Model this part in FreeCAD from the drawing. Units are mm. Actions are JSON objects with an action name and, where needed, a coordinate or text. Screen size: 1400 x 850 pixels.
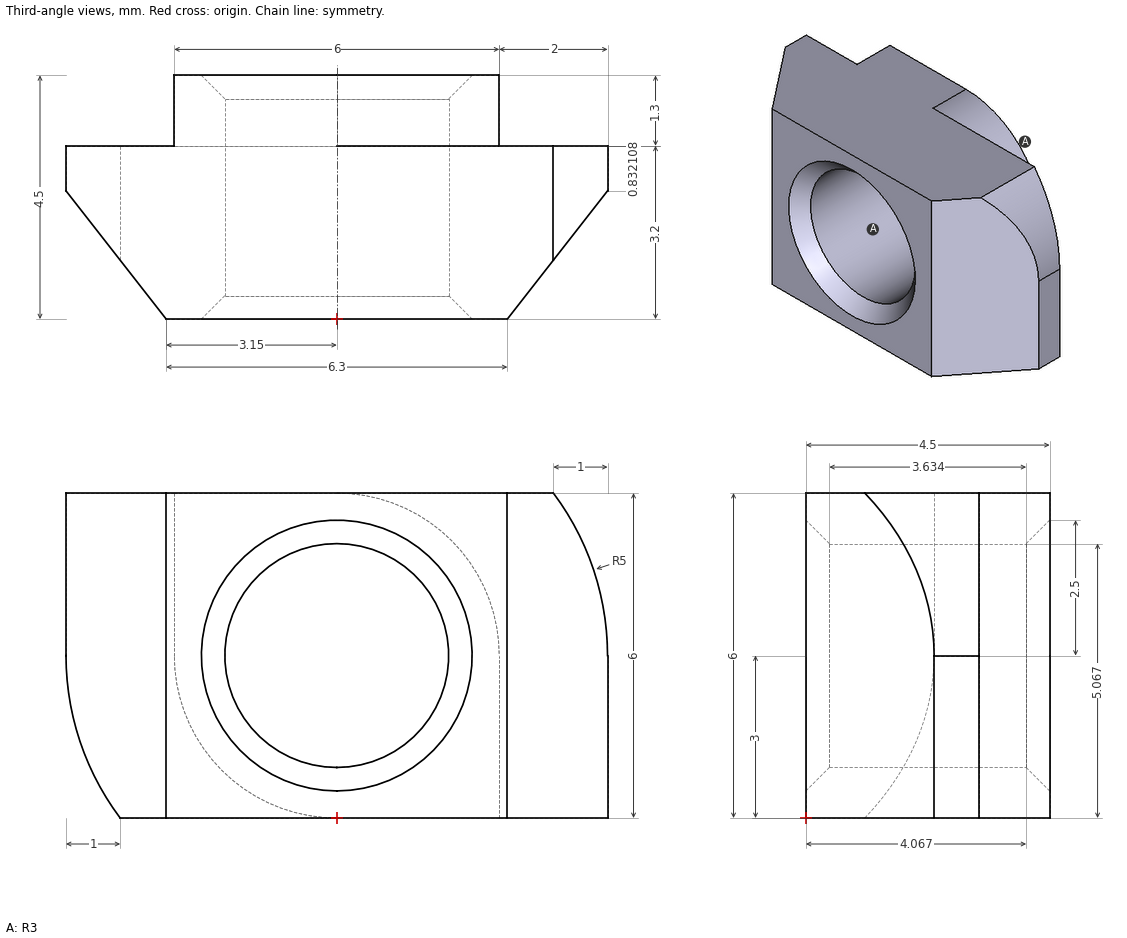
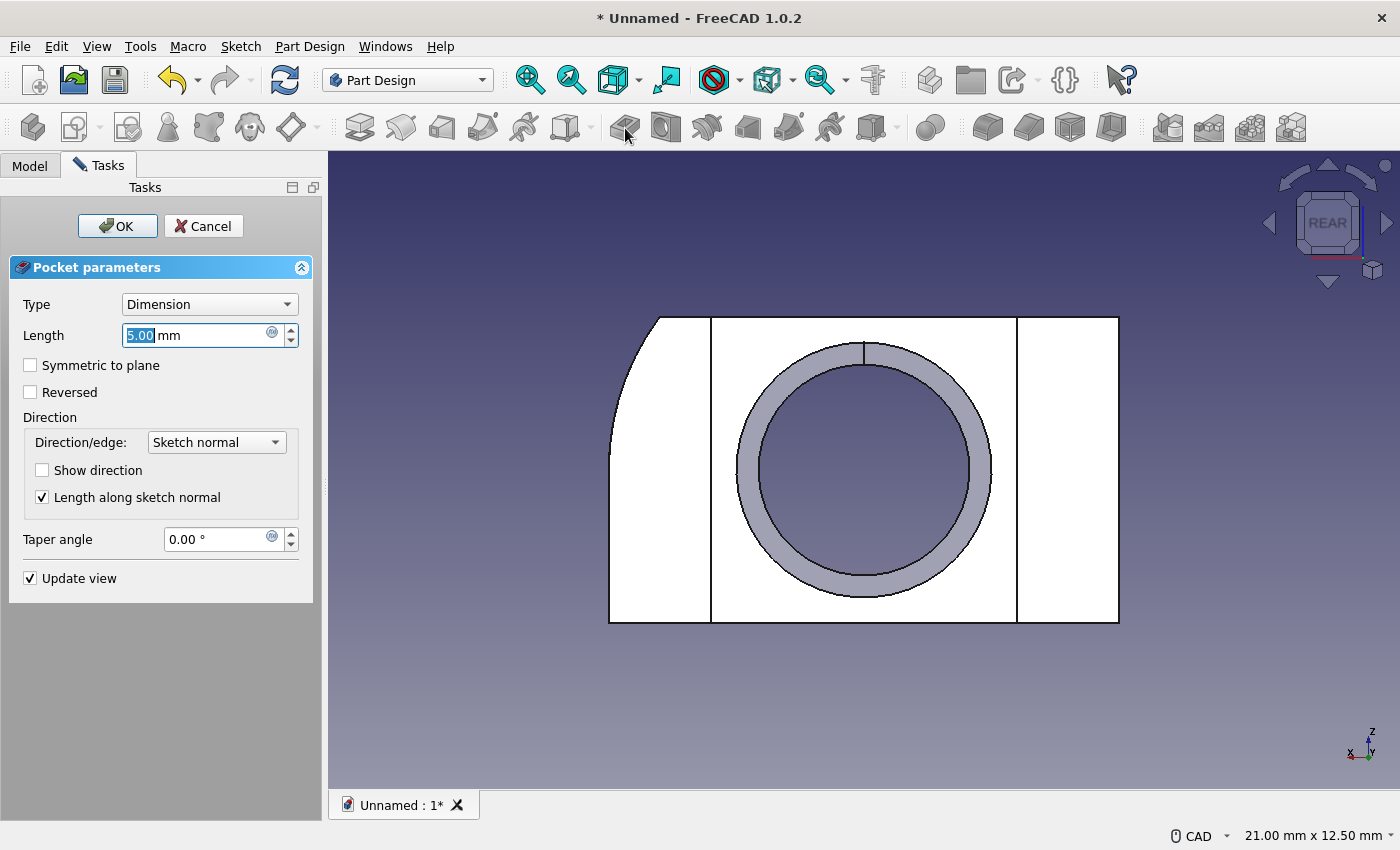
{"action": "type", "text": "4.5"}
{"action": "key", "text": "Tab"}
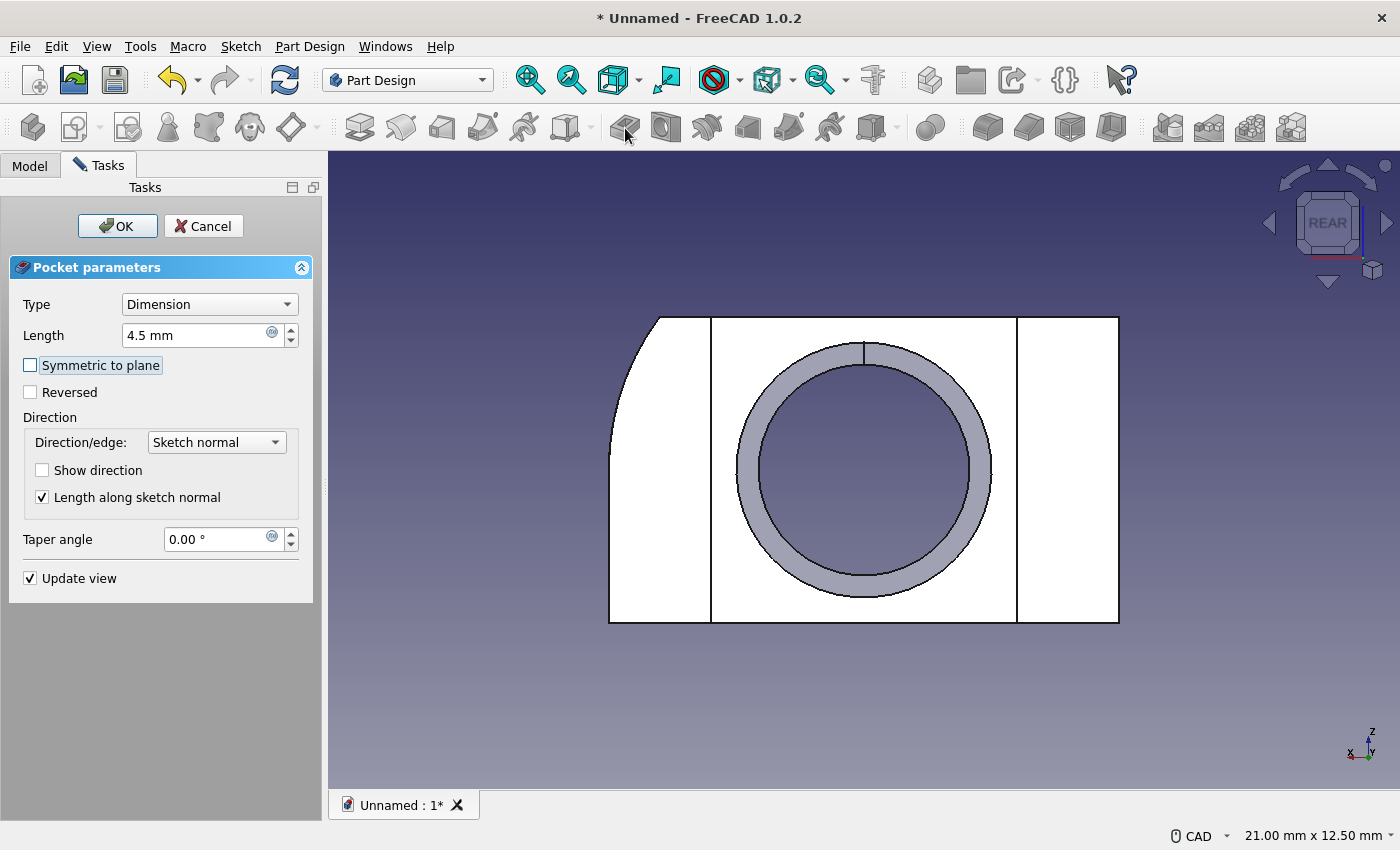
{"action": "left_click", "coordinate": [118, 226]}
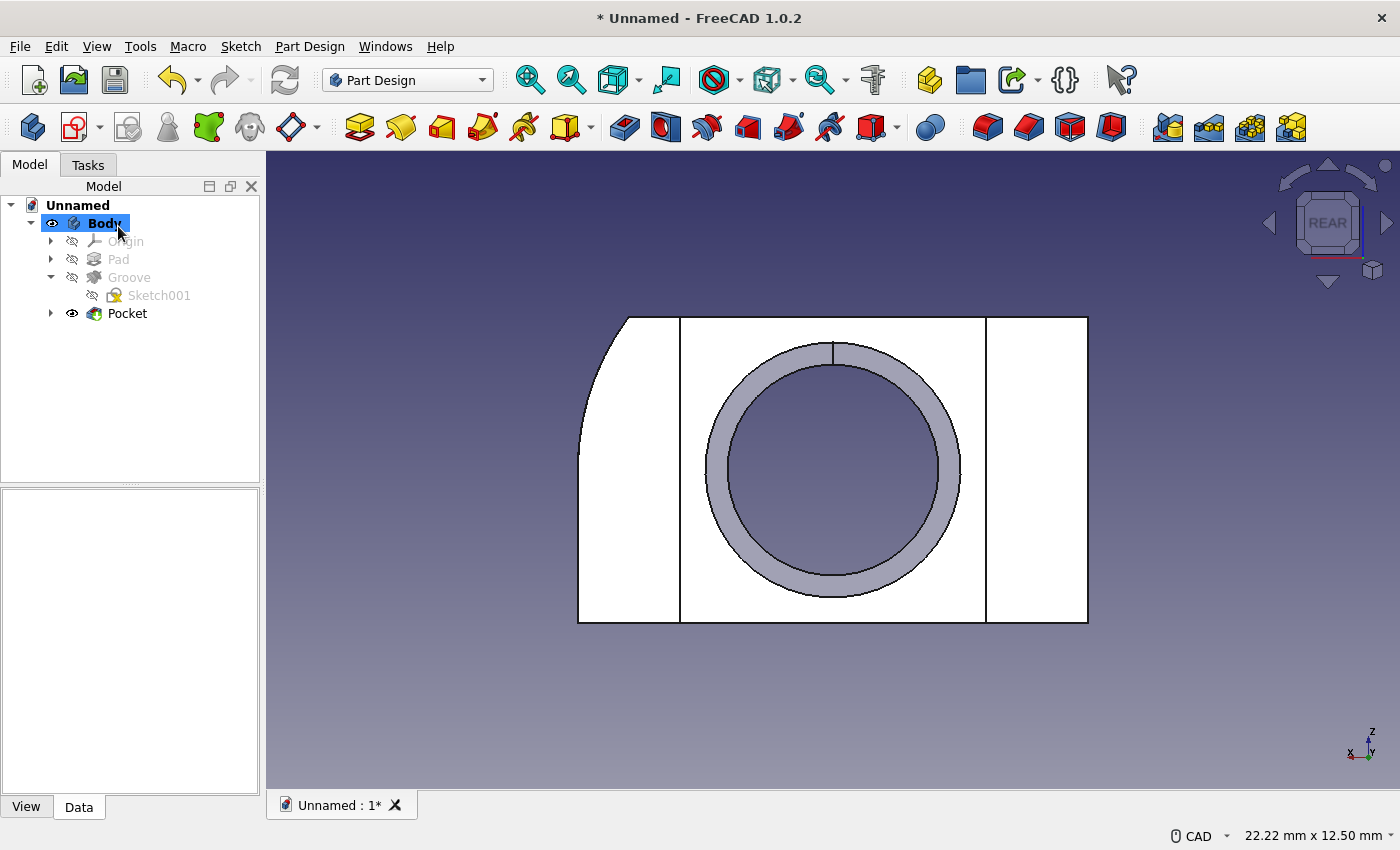
{"action": "left_click", "coordinate": [746, 338]}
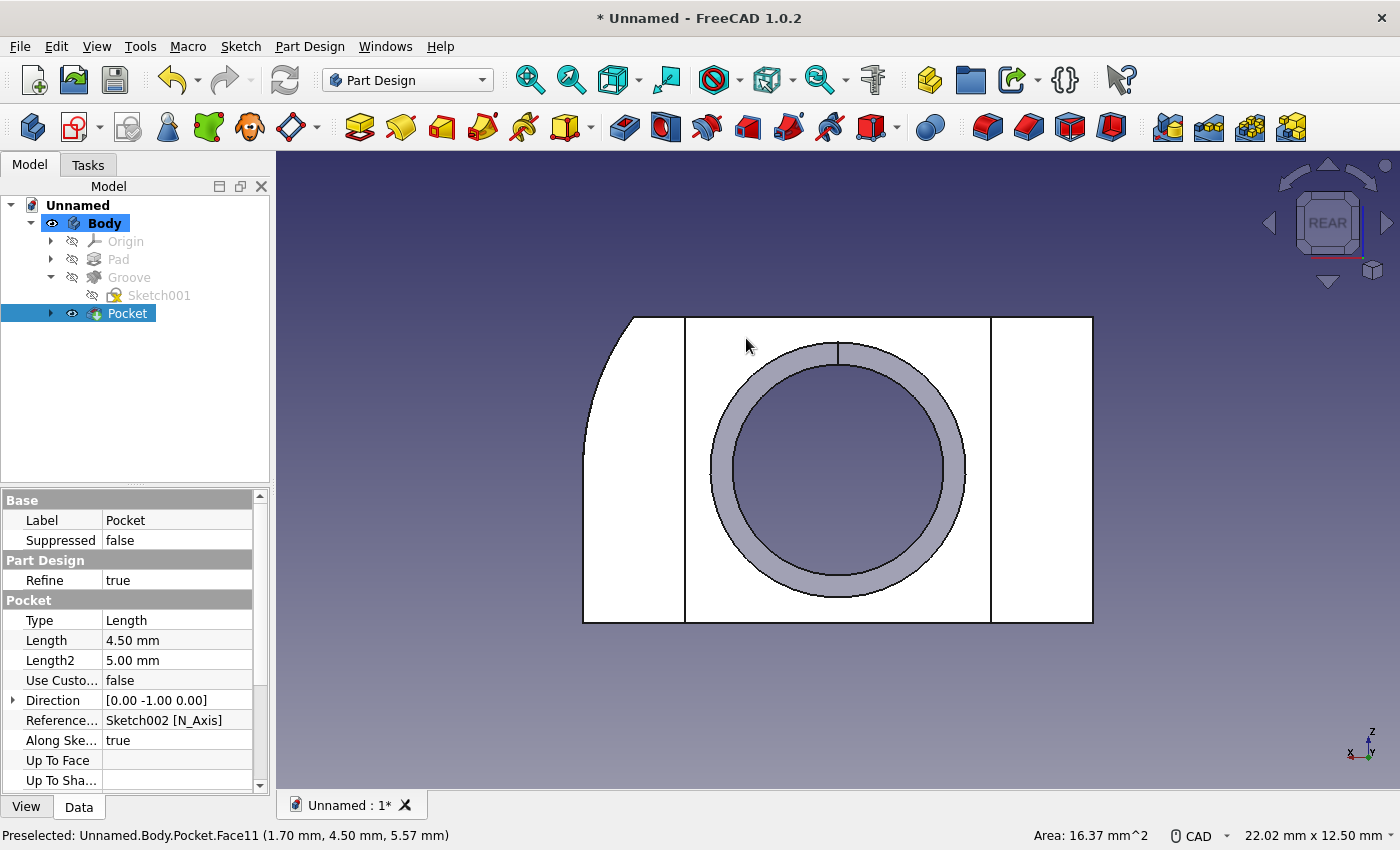
{"action": "left_click", "coordinate": [74, 128]}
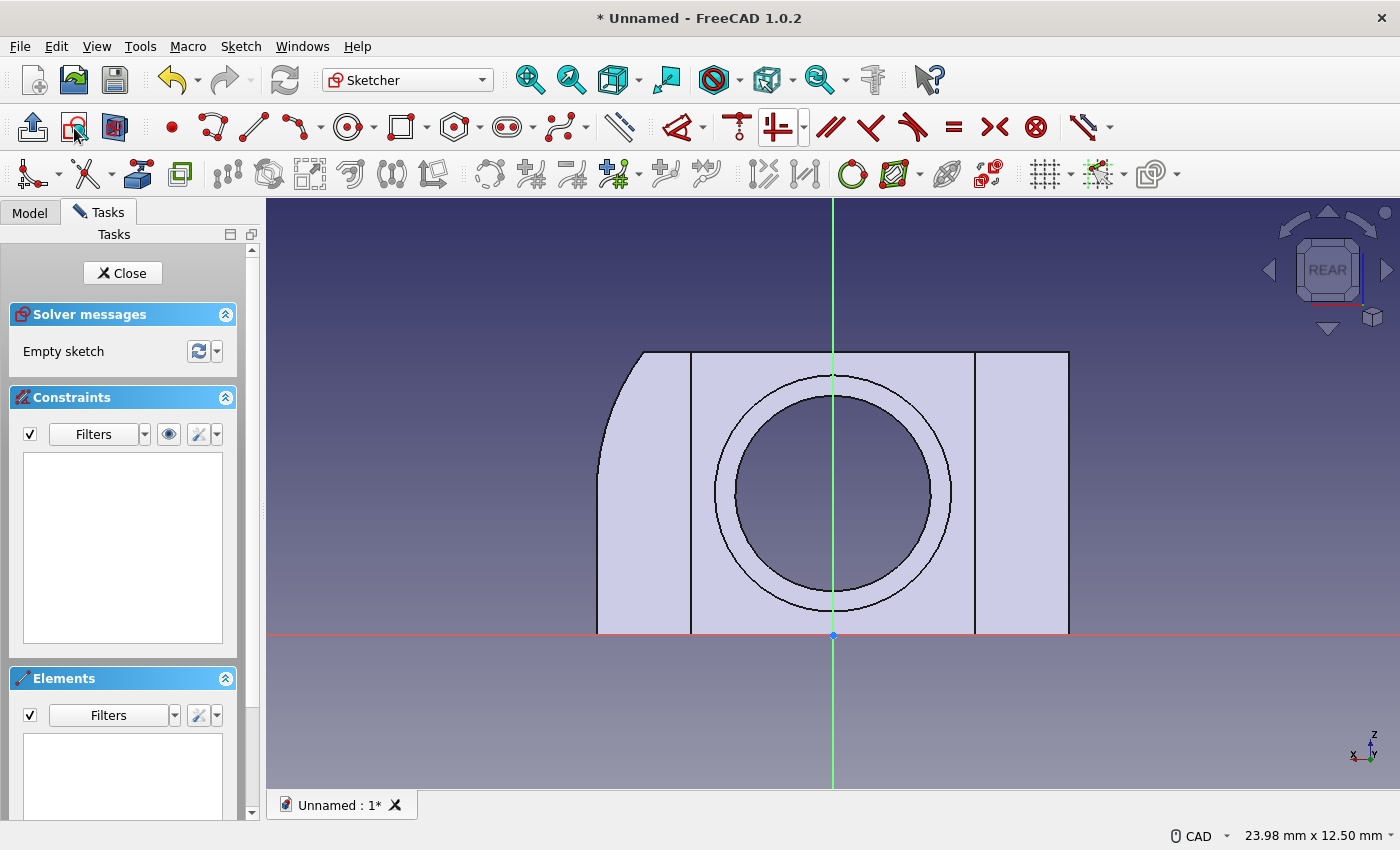
{"action": "scroll", "coordinate": [1060, 606], "scroll_direction": "up", "scroll_amount": 5}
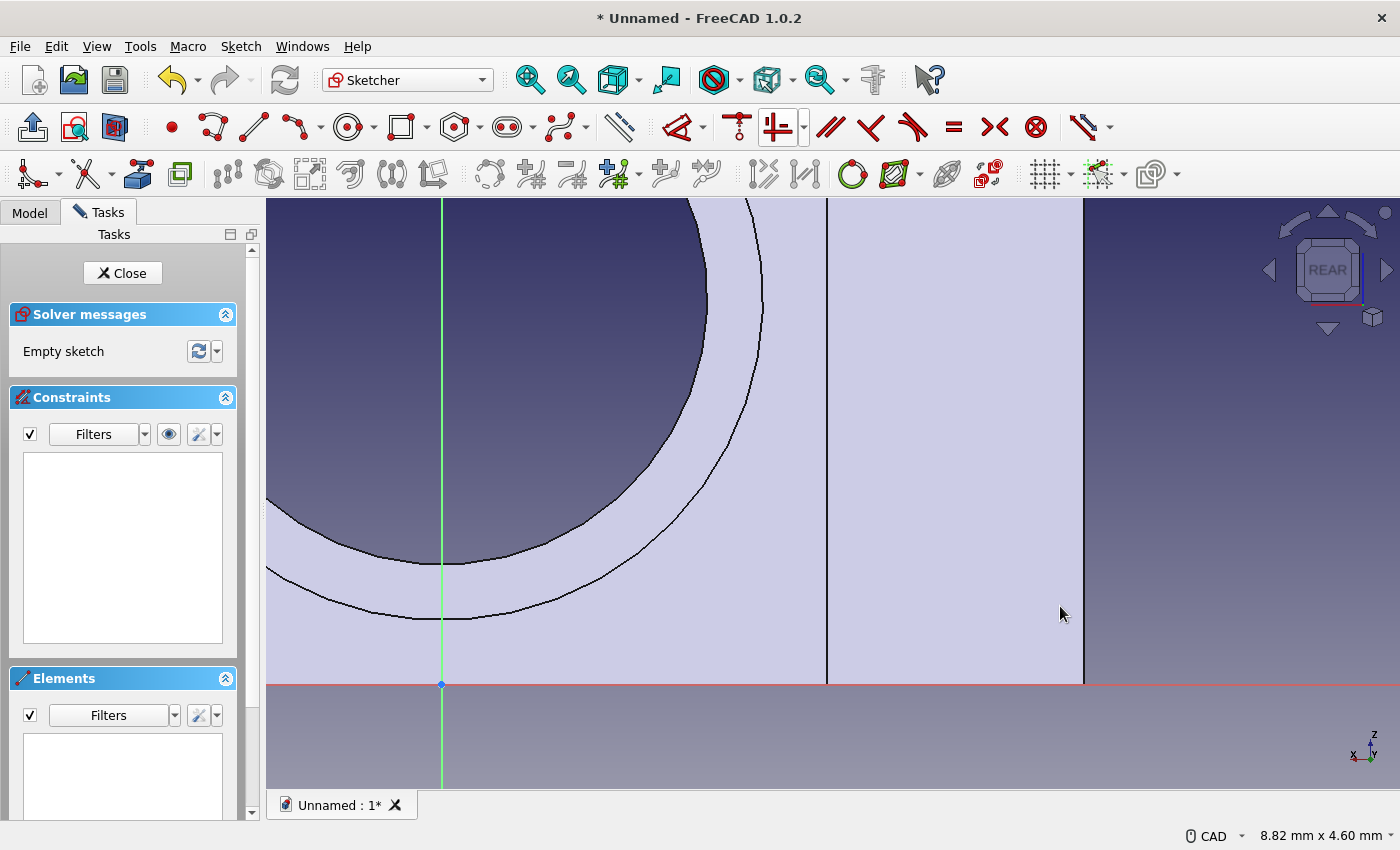
{"action": "left_click", "coordinate": [213, 128]}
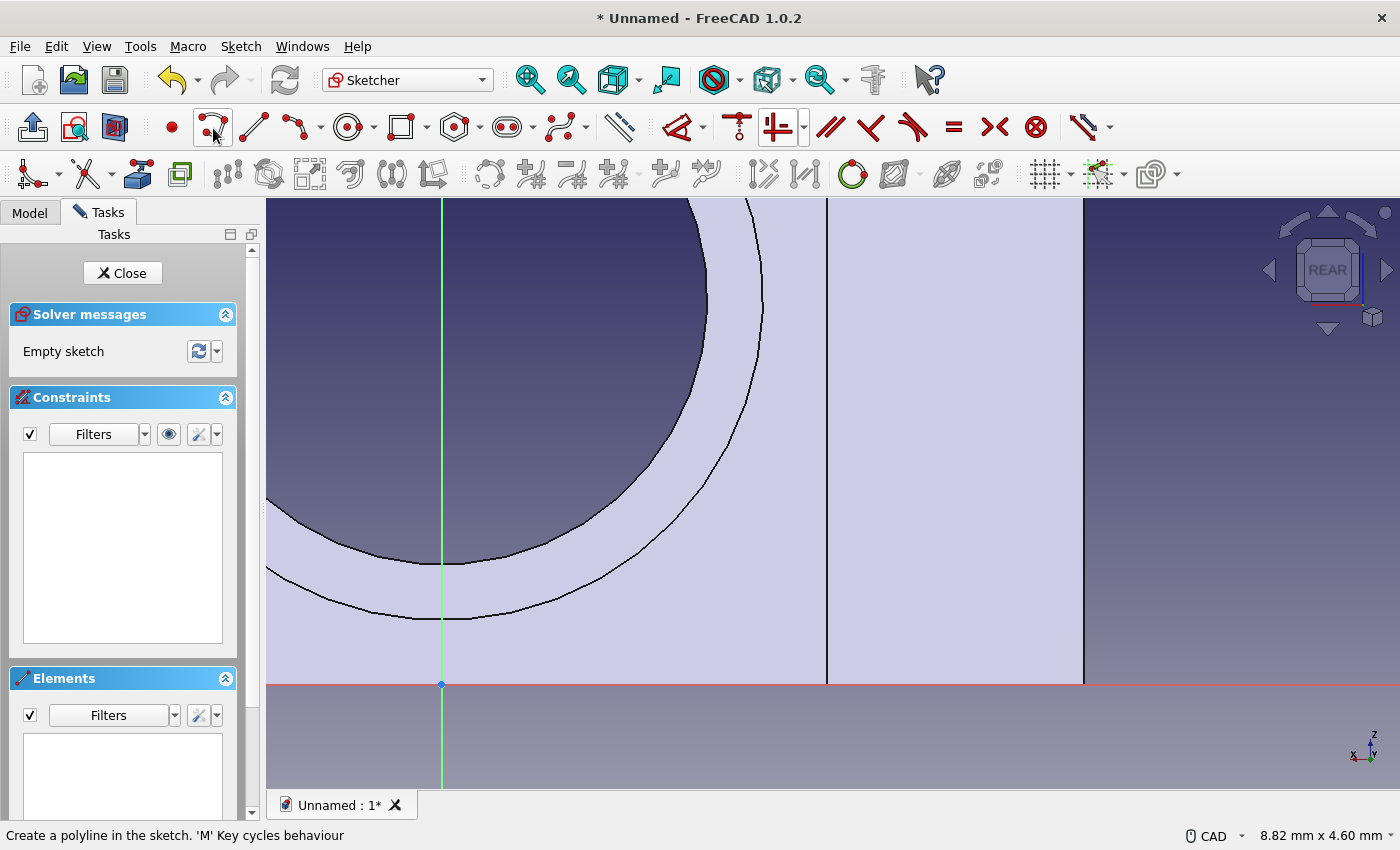
{"action": "left_click", "coordinate": [956, 685]}
{"action": "left_click", "coordinate": [1084, 676]}
{"action": "left_click", "coordinate": [1084, 299]}
{"action": "right_click", "coordinate": [1084, 299]}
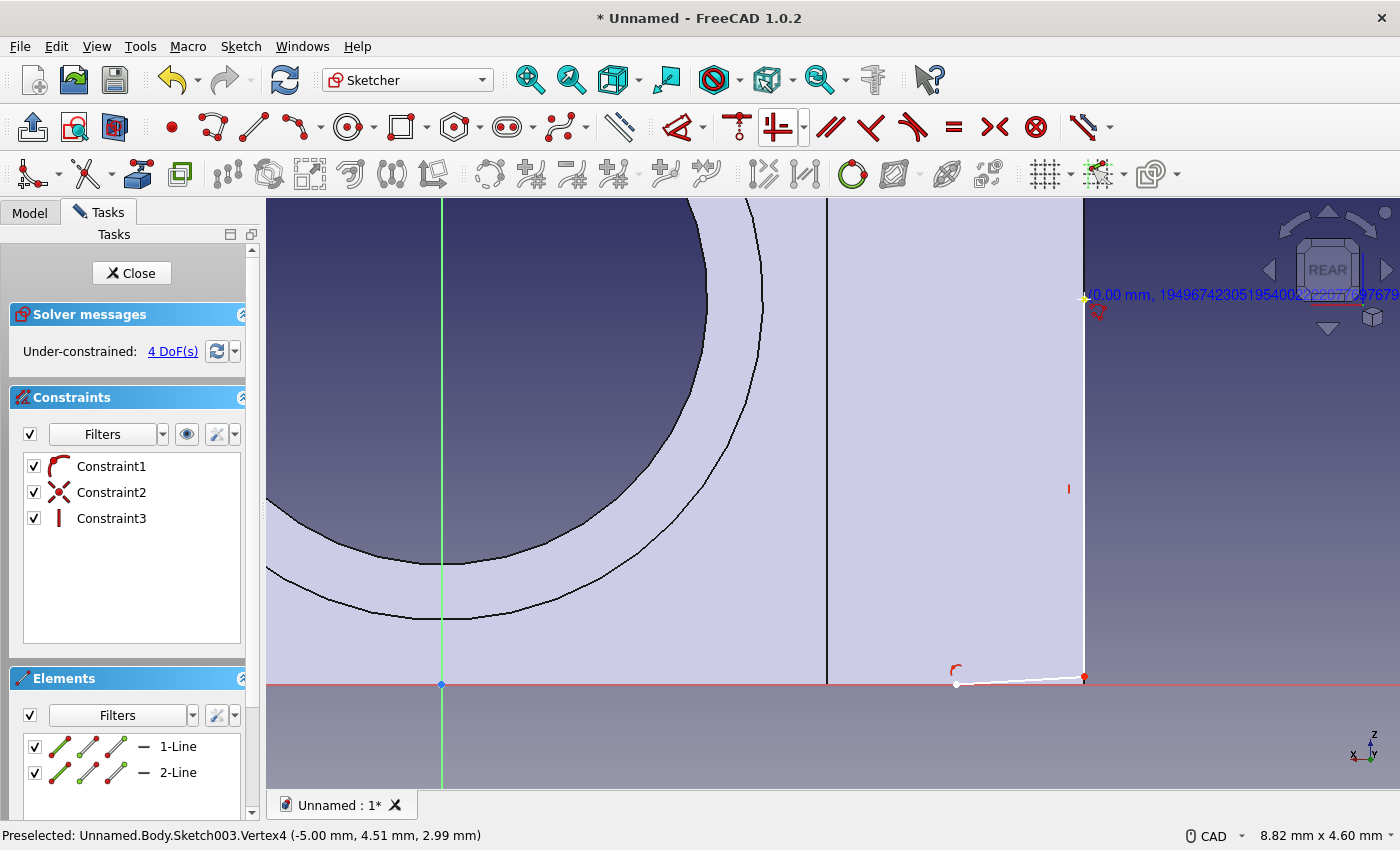
{"action": "left_click", "coordinate": [294, 128]}